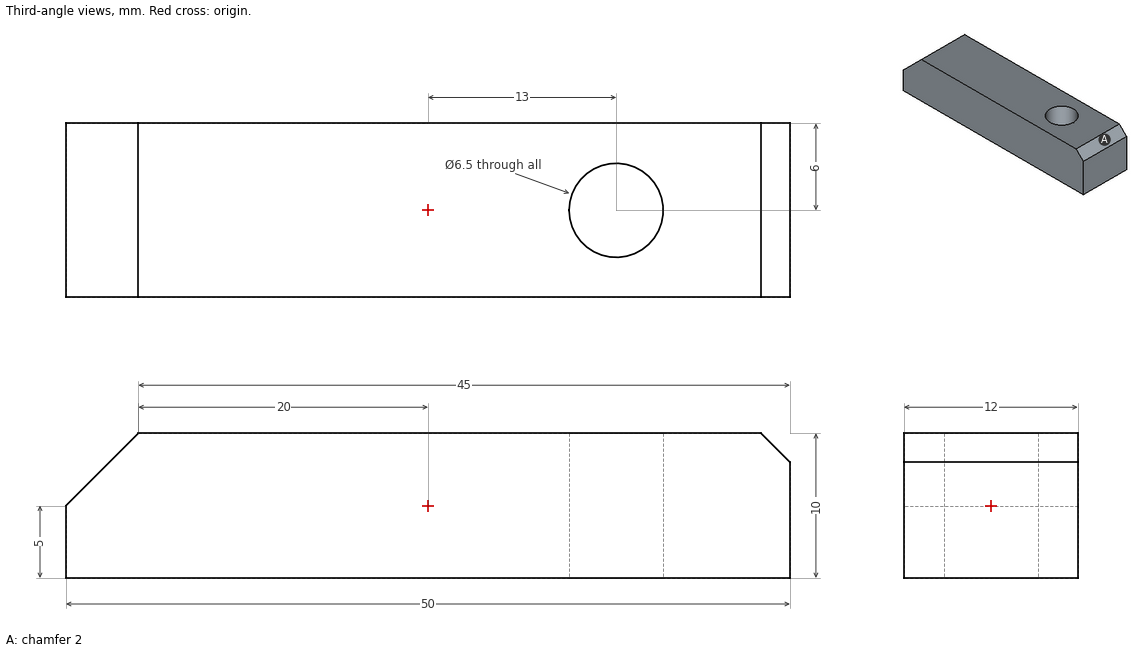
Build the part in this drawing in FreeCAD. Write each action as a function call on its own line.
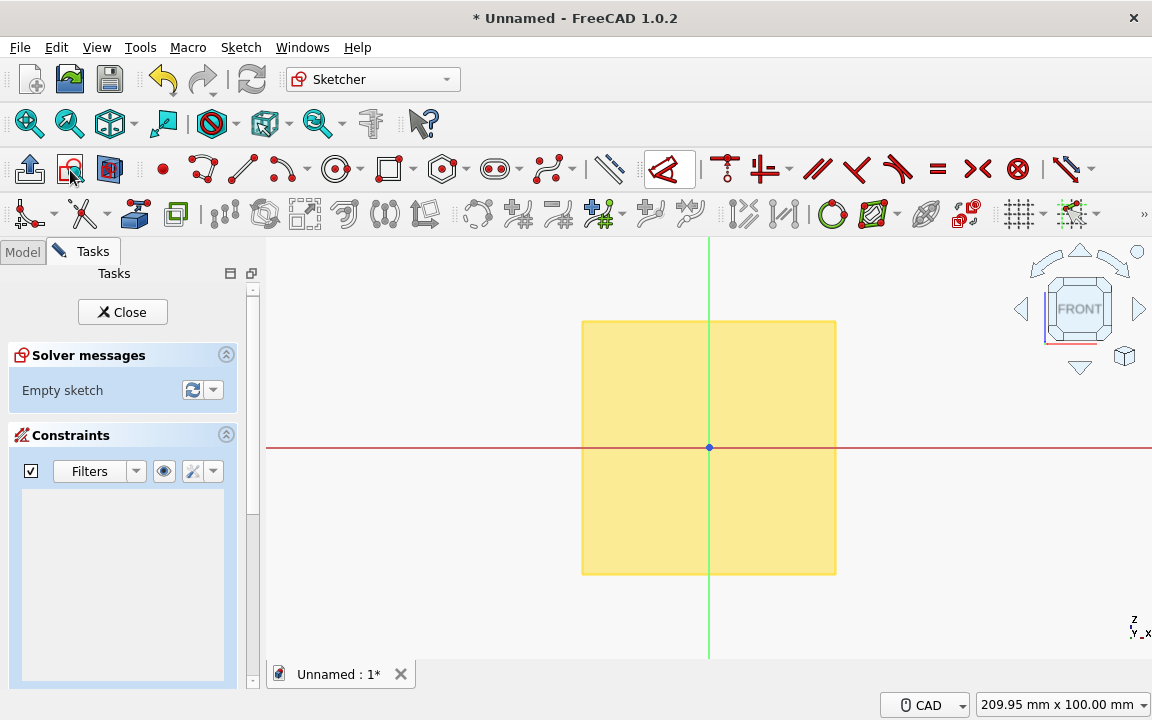
scroll(765, 448, up, 4)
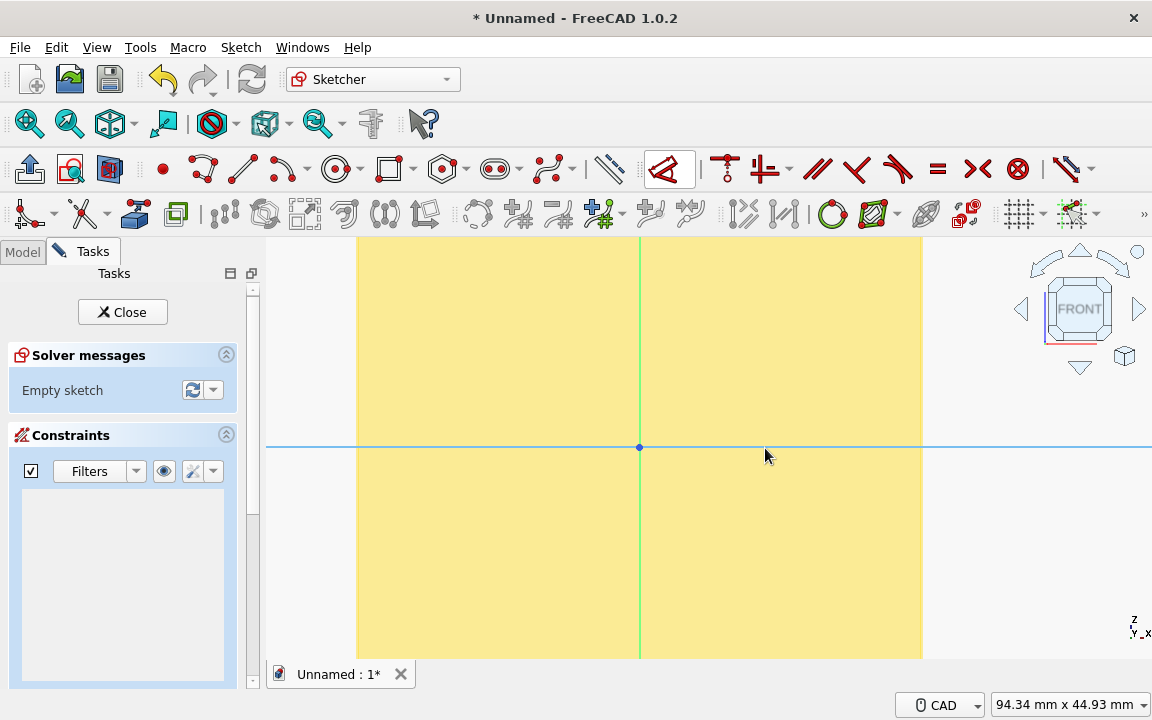
click(204, 170)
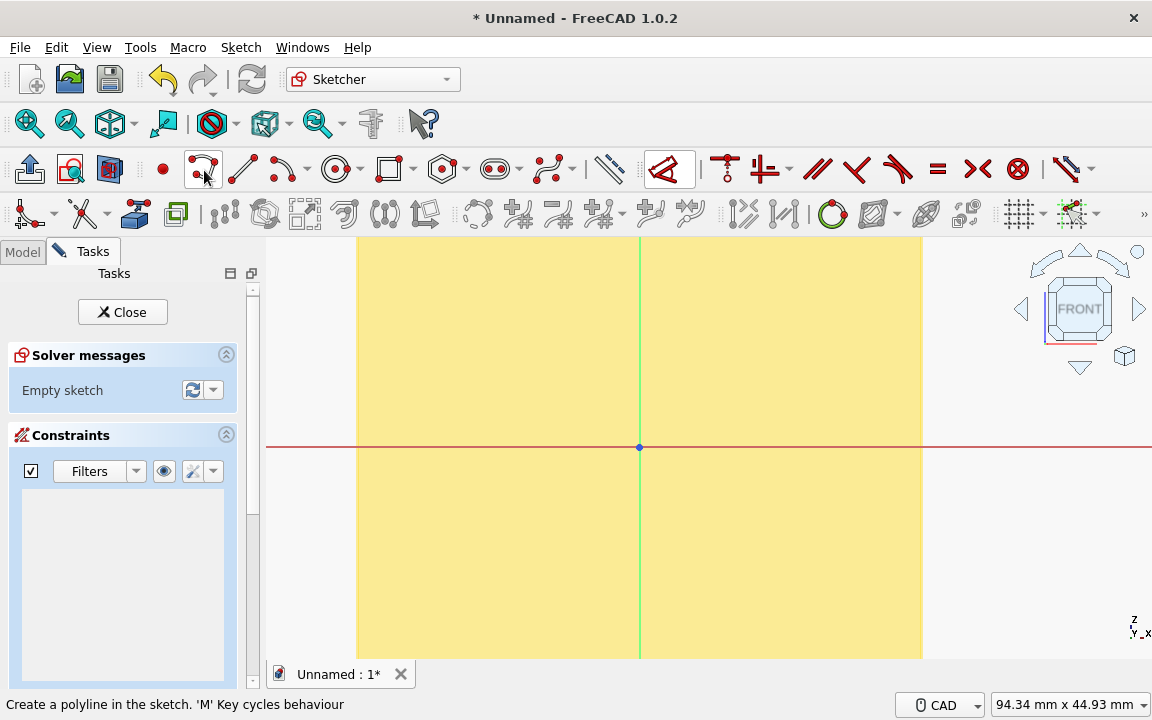
click(452, 400)
click(874, 400)
click(874, 494)
click(405, 494)
click(405, 447)
click(452, 401)
key(Escape)
key(Escape)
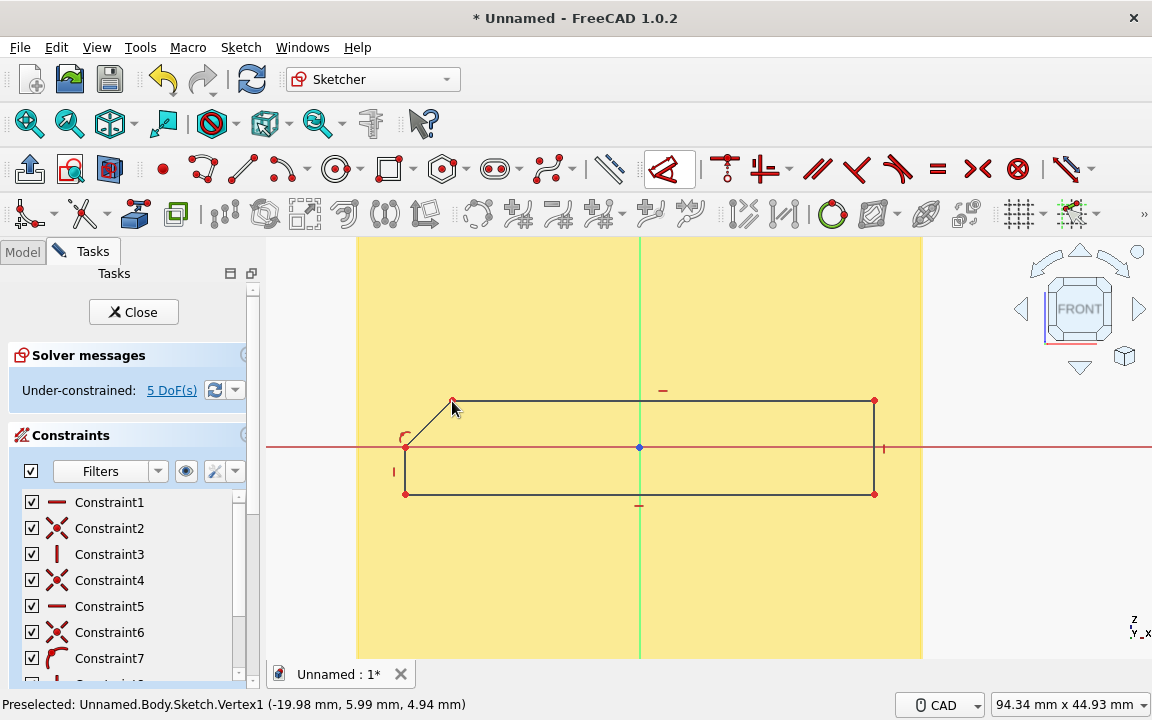
click(405, 481)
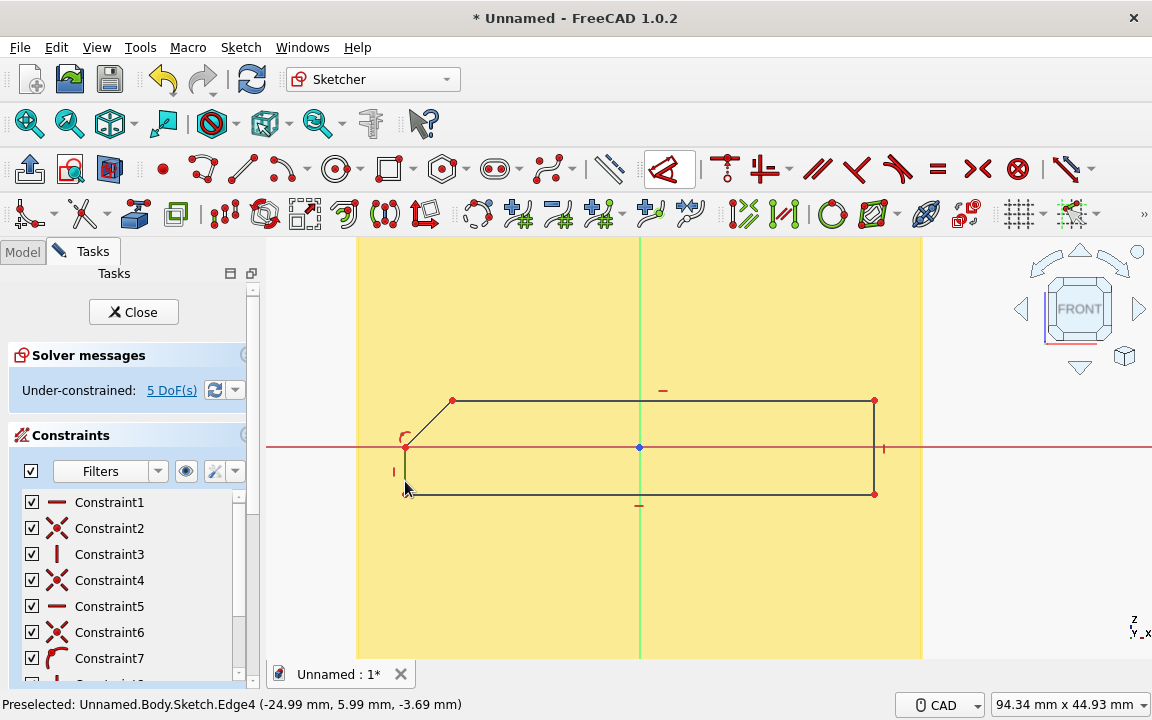
key(i)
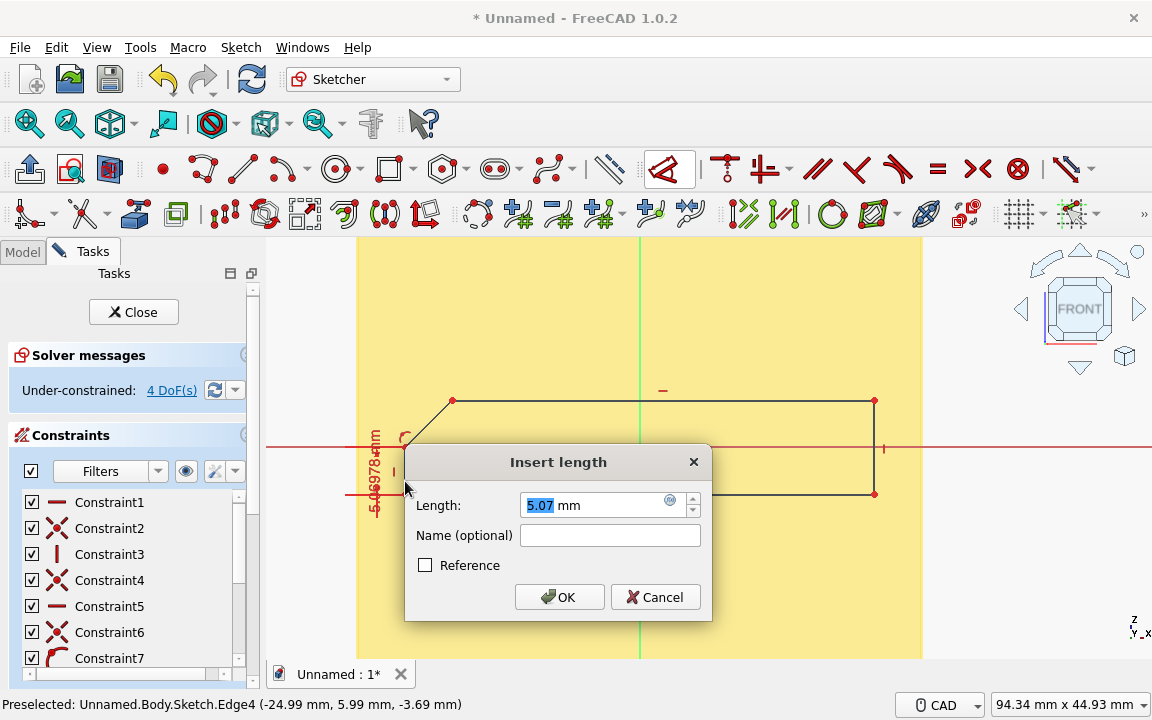
text(5)
key(Return)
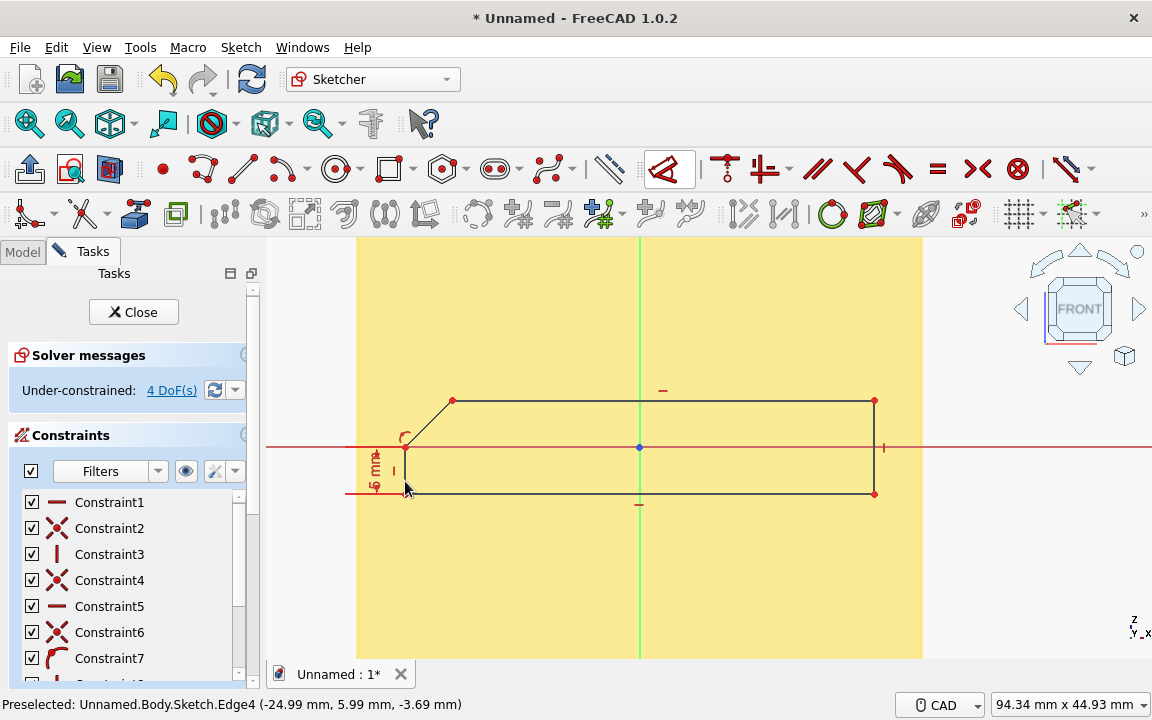
click(579, 401)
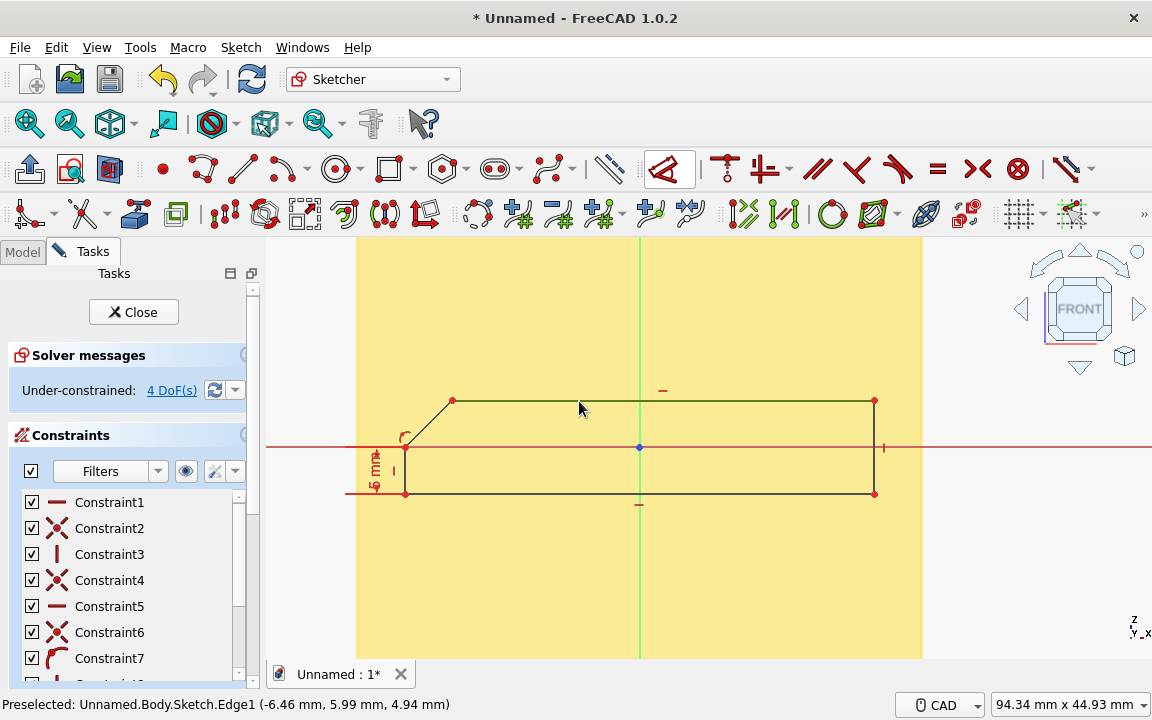
click(690, 170)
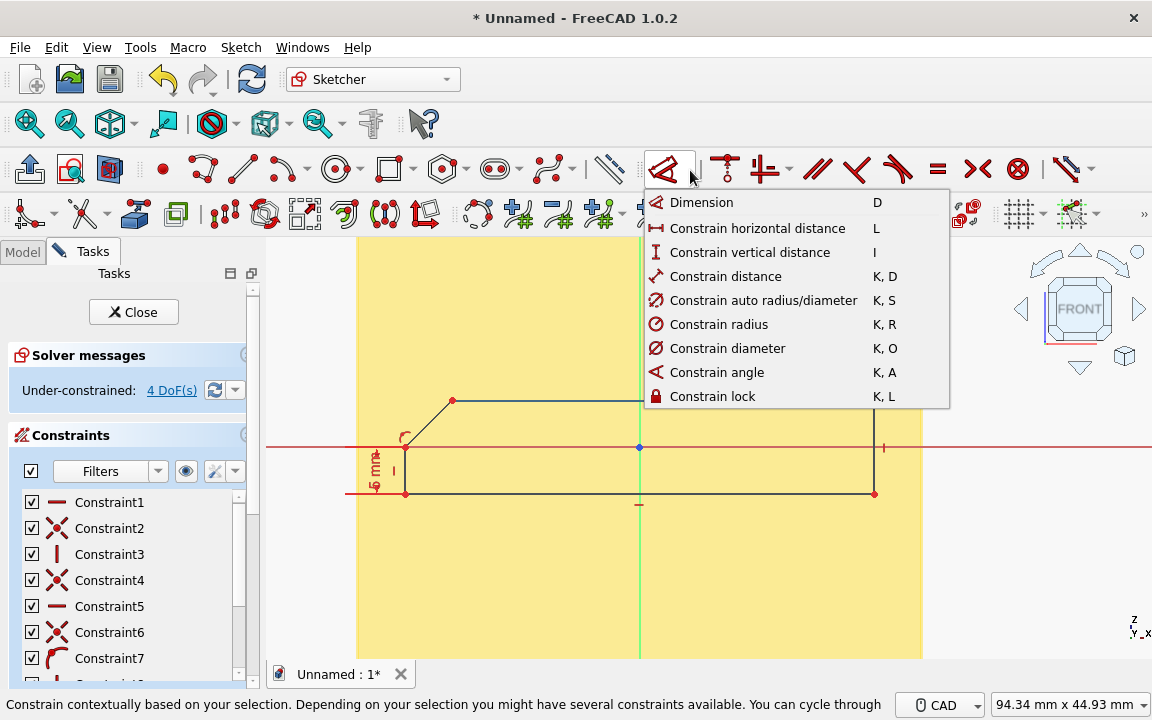
click(797, 228)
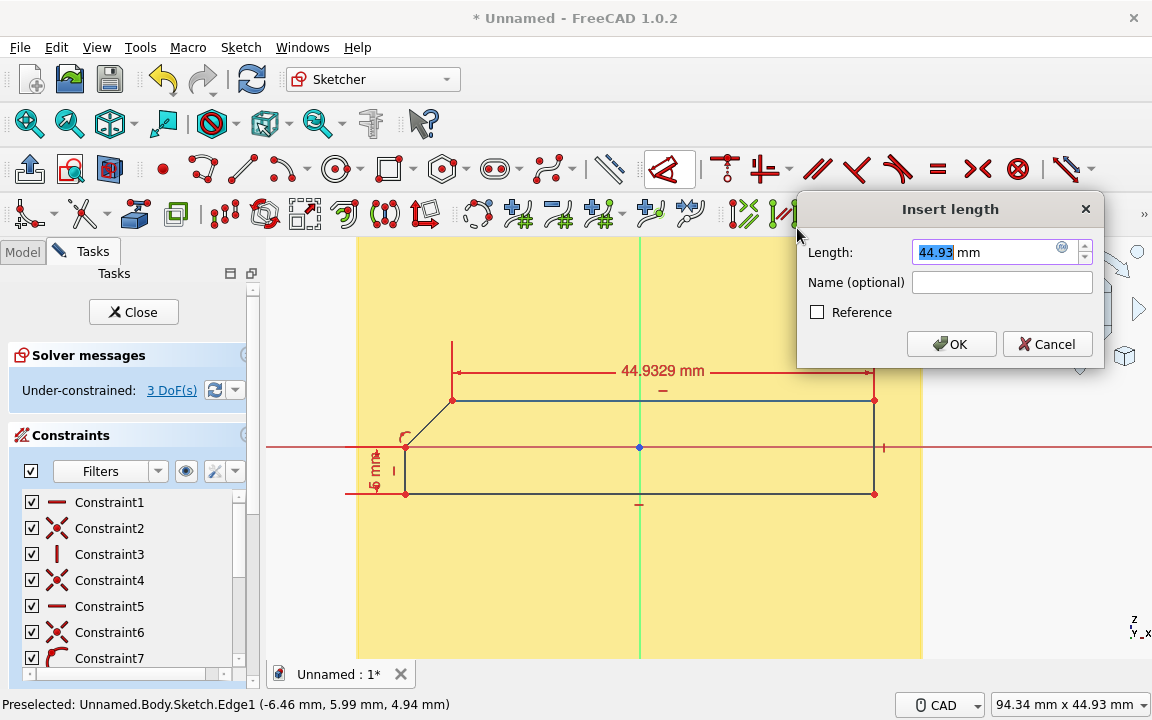
text(45)
key(Return)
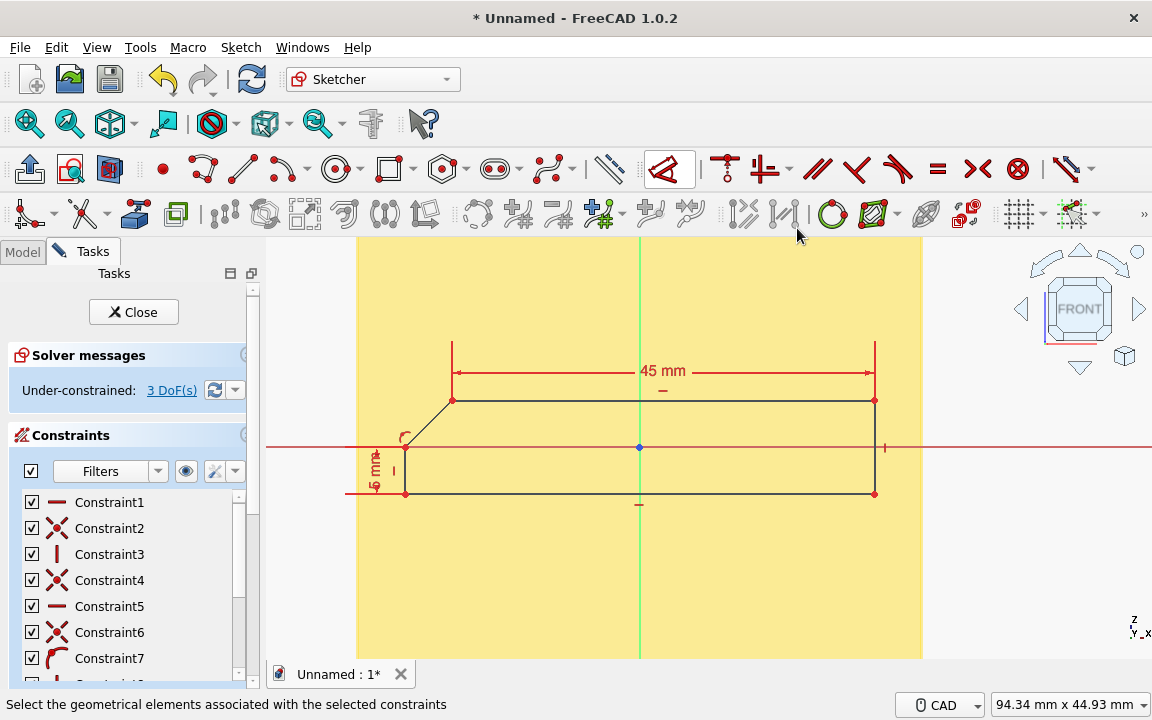
click(875, 429)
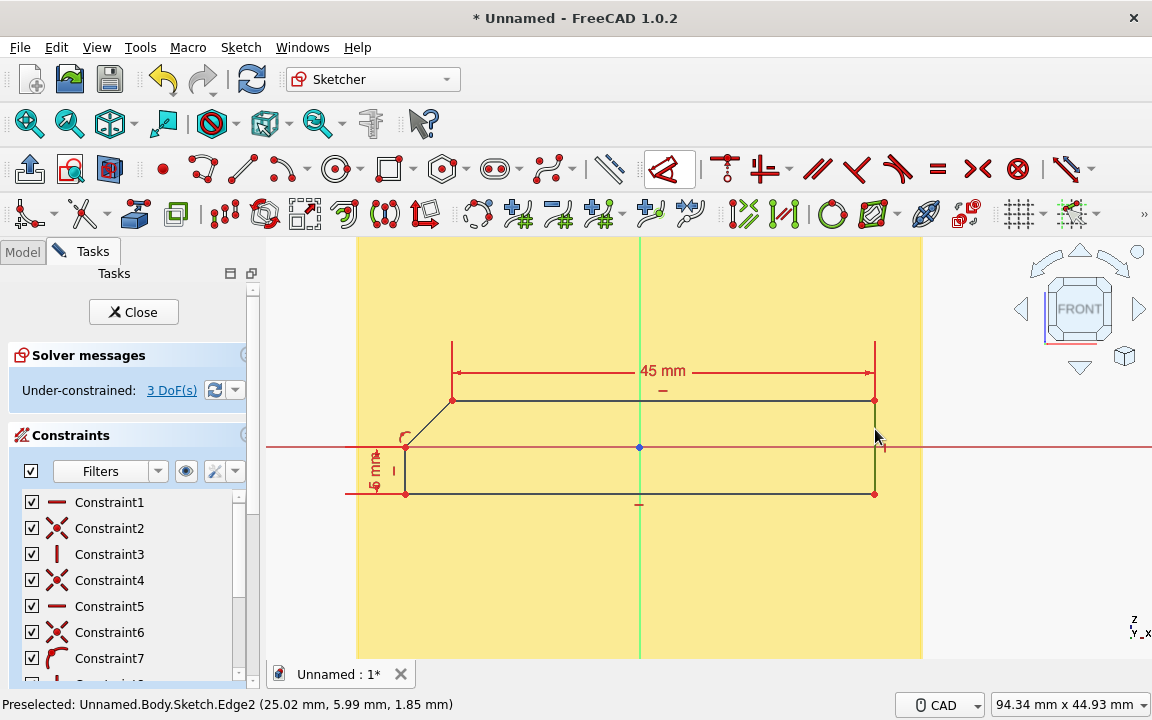
key(i)